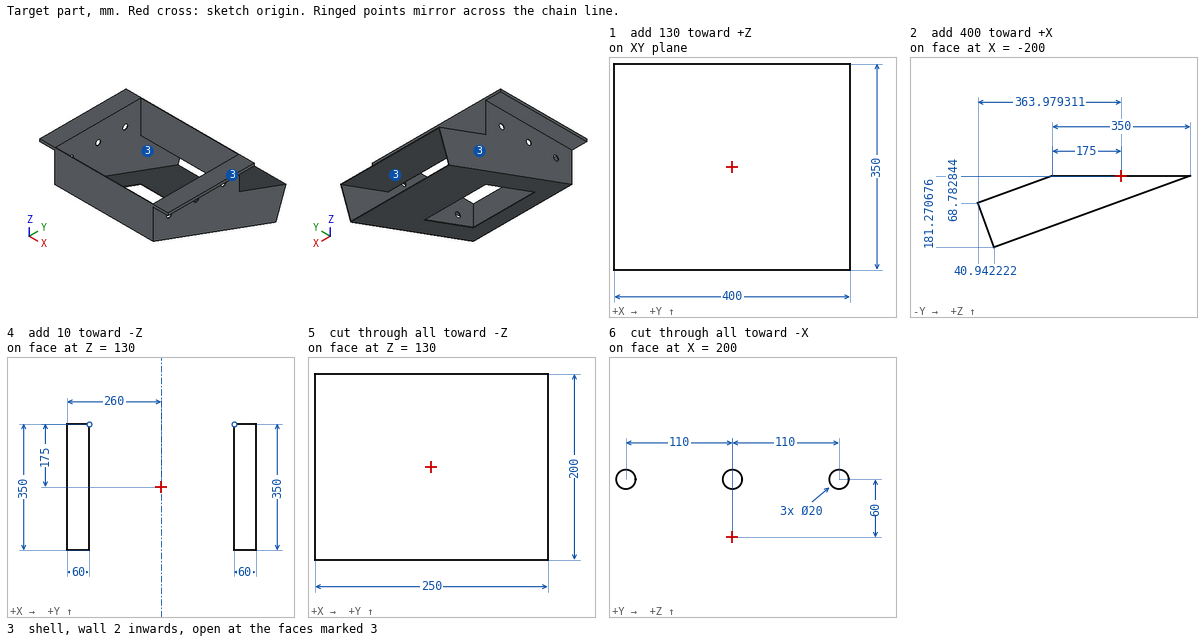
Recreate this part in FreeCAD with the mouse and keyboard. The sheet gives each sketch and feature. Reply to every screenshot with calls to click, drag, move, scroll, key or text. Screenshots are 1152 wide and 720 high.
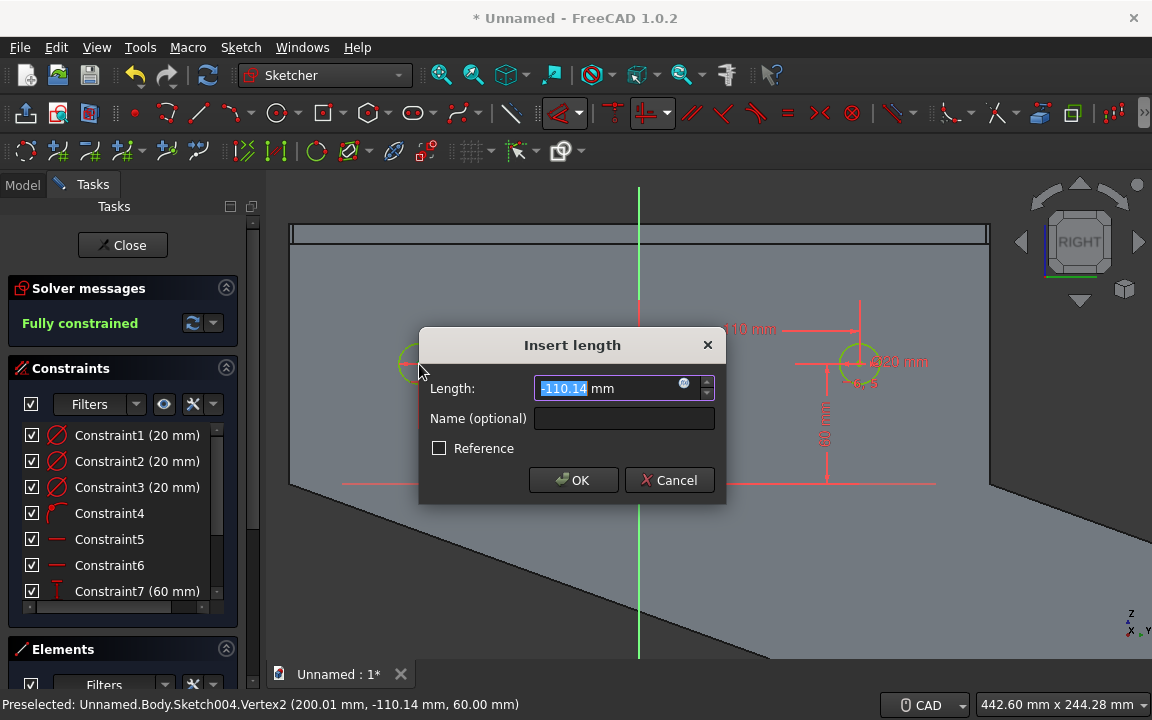
text(-110)
key(Return)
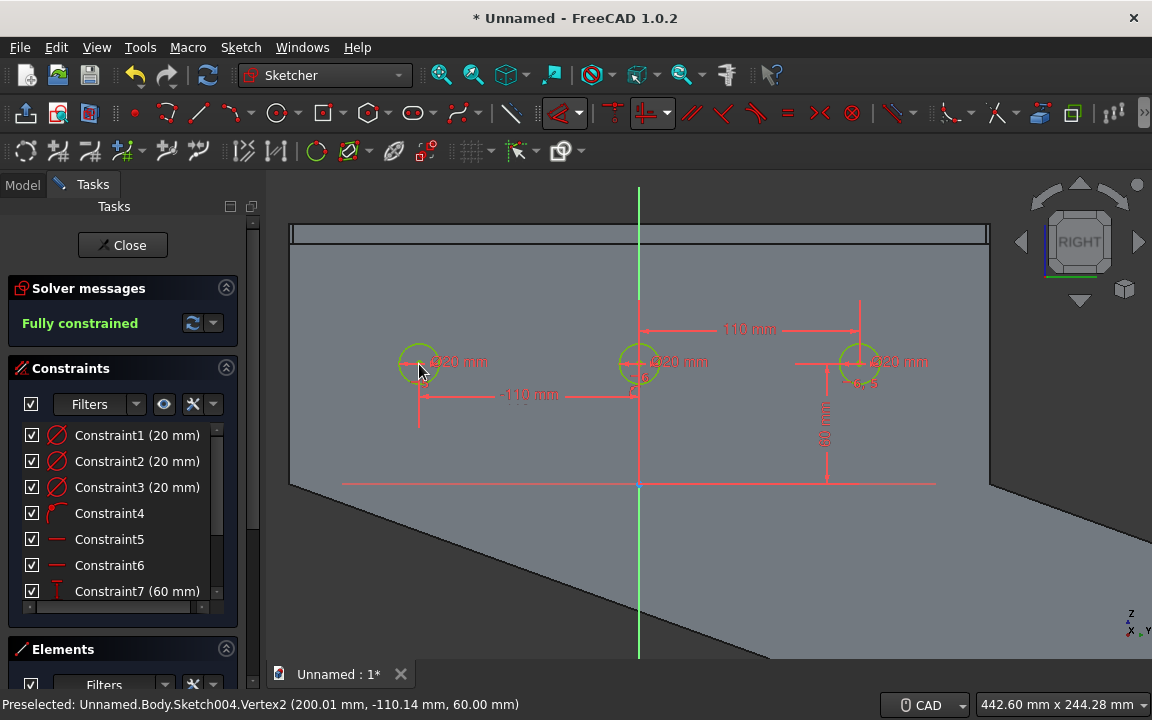
click(123, 245)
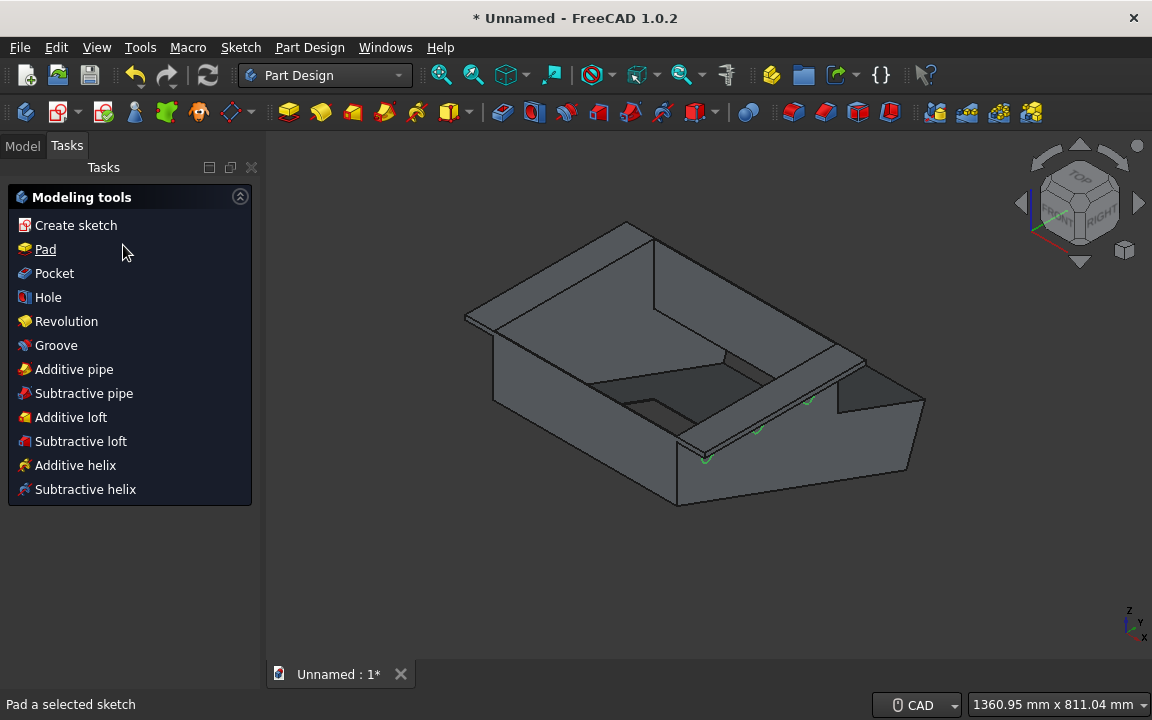
click(504, 112)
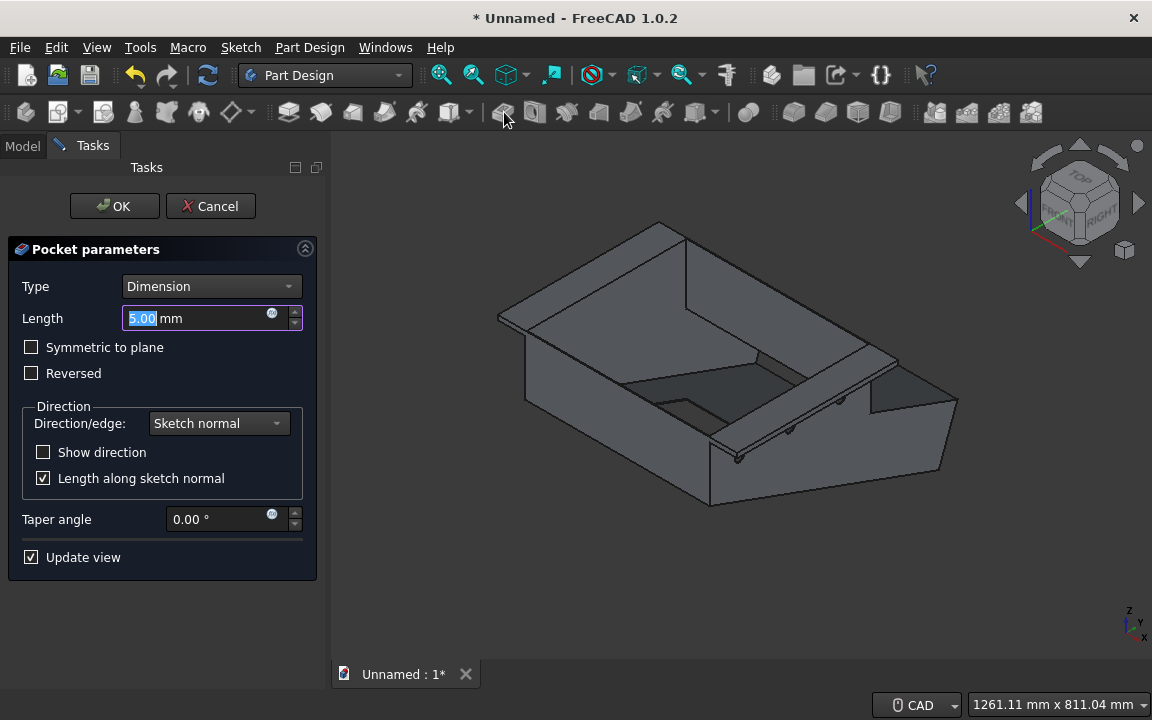
click(212, 286)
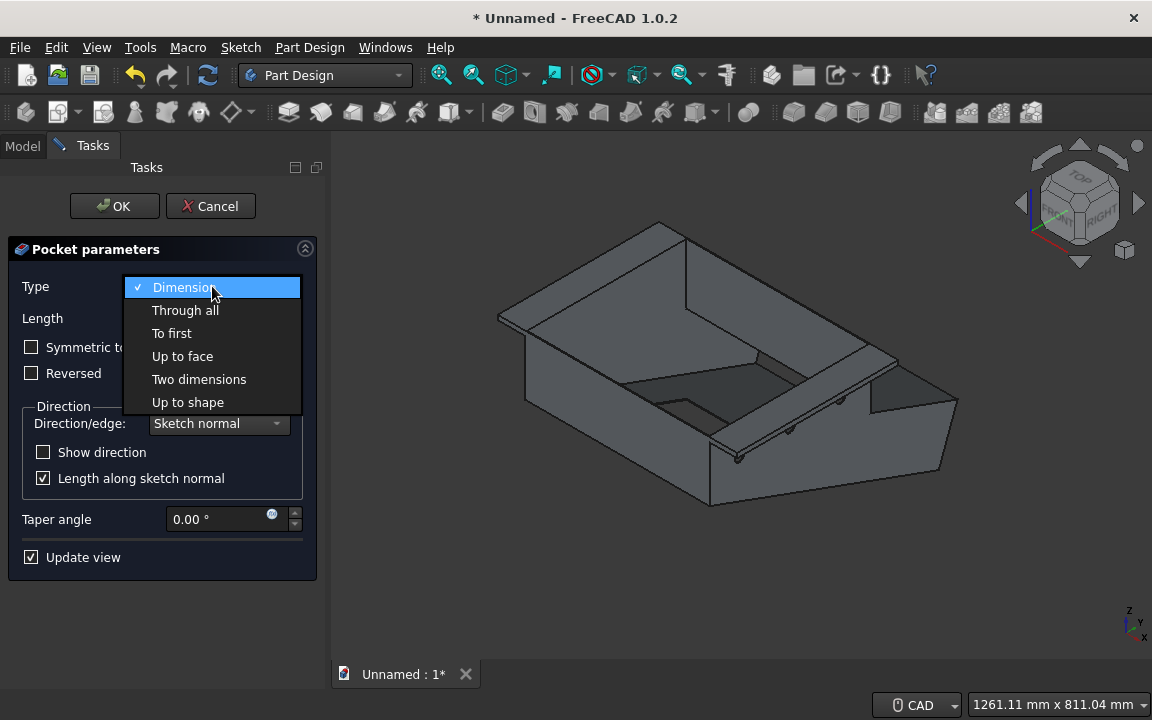
click(212, 310)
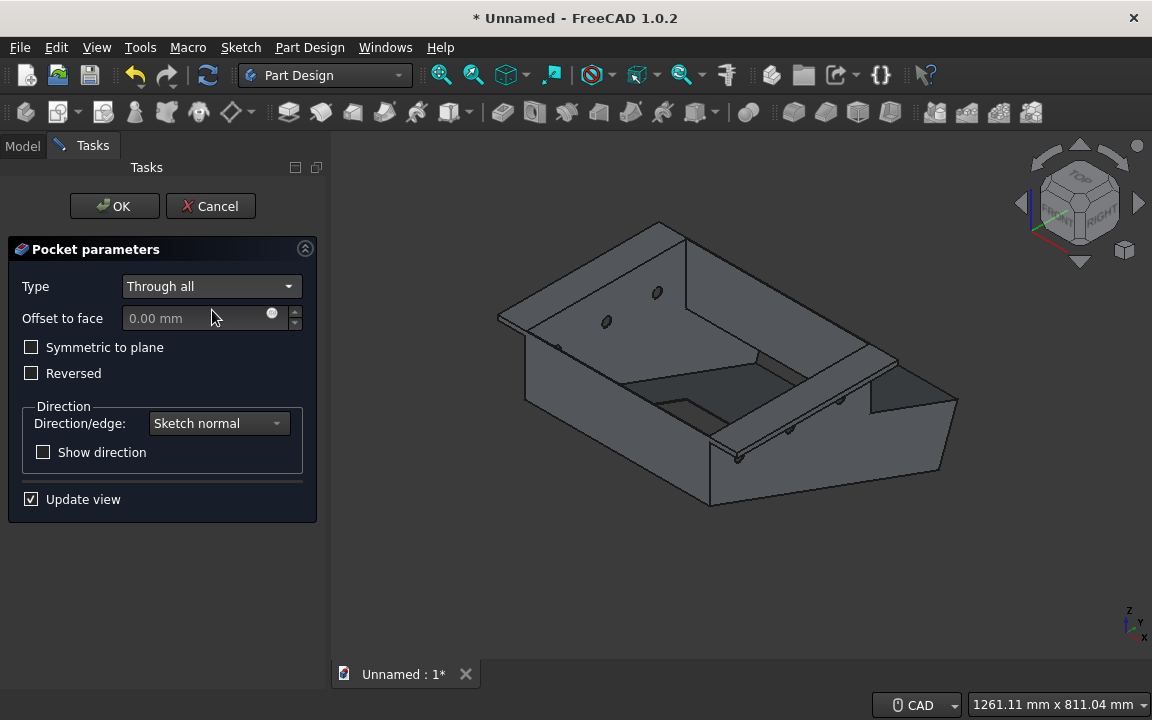
click(115, 206)